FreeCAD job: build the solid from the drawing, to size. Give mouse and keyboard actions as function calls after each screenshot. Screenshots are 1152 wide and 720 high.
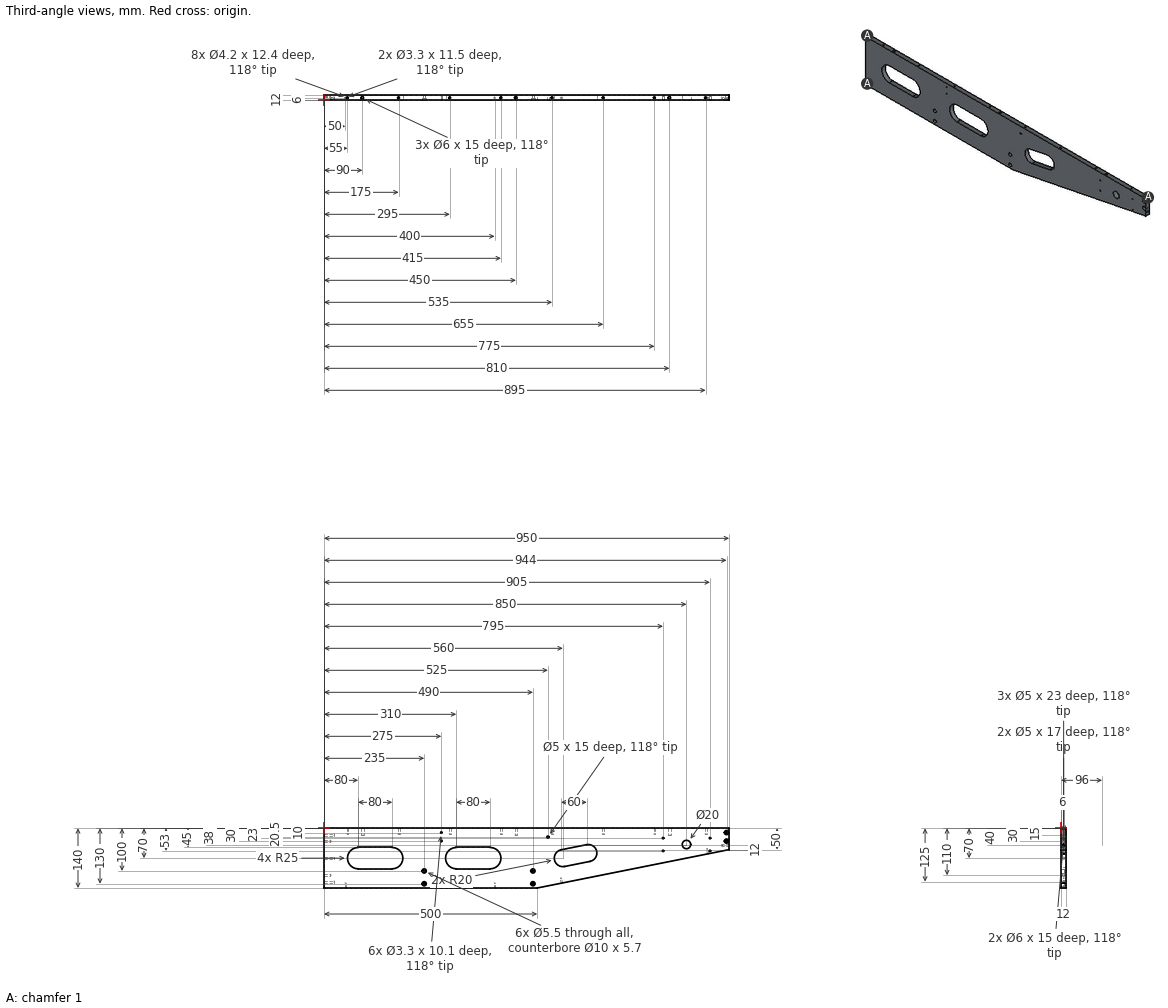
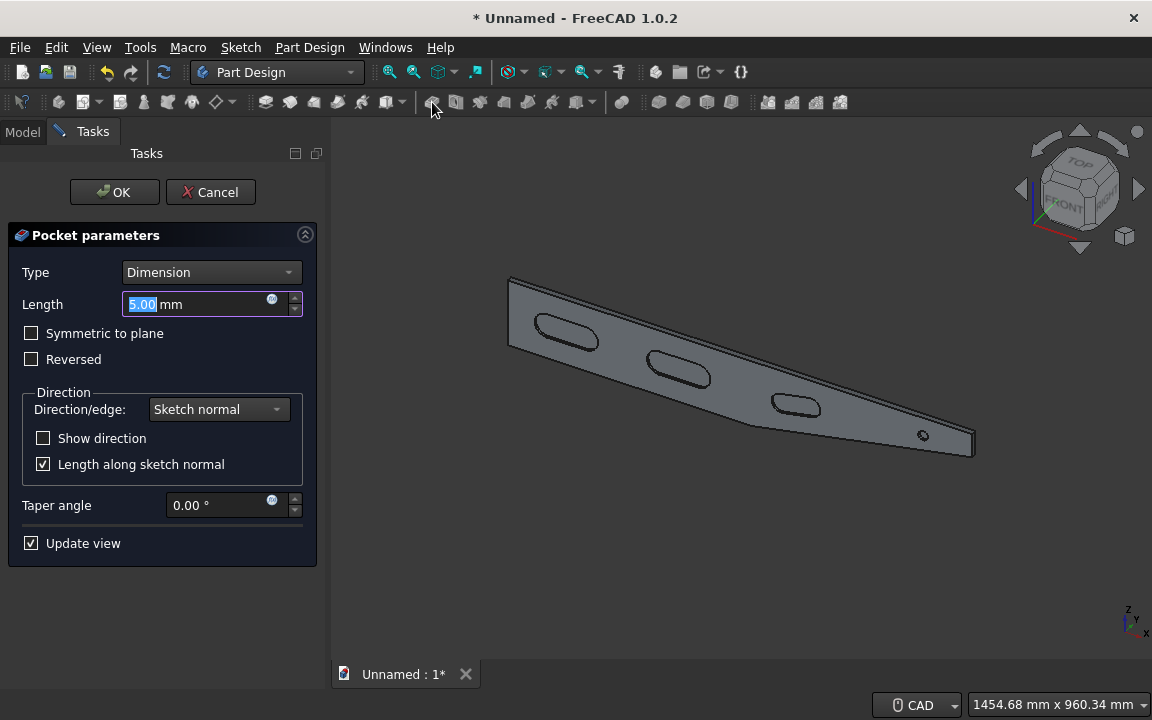
text(12)
key(Tab)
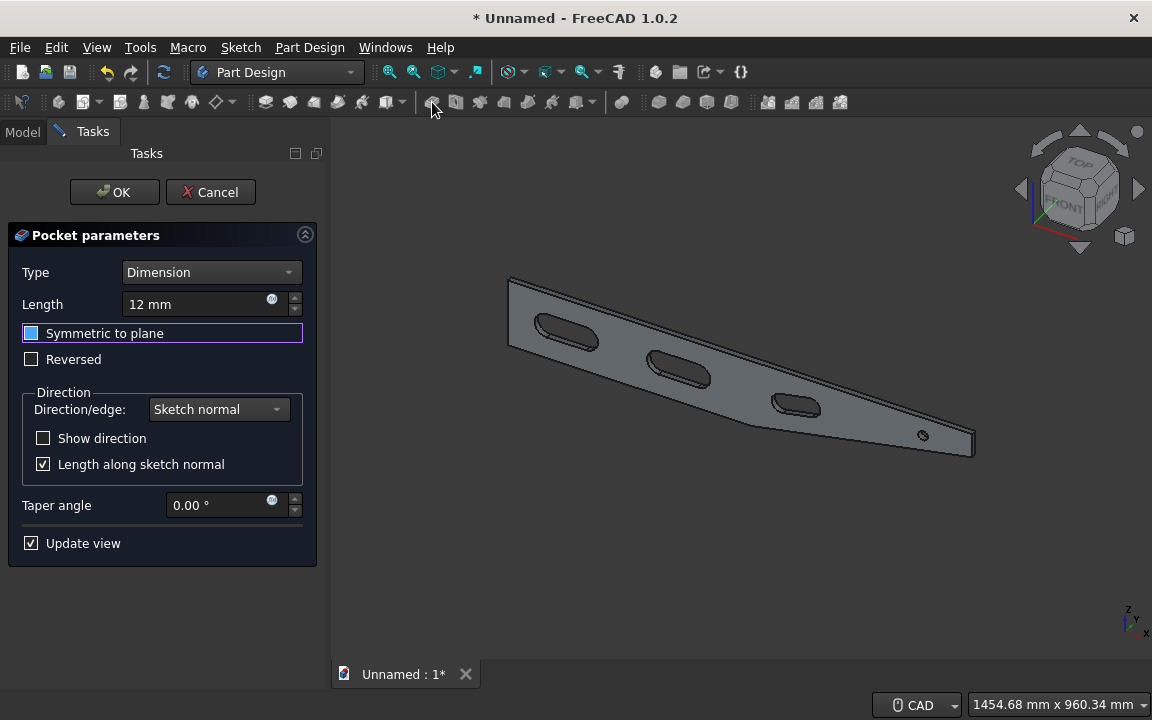
click(115, 192)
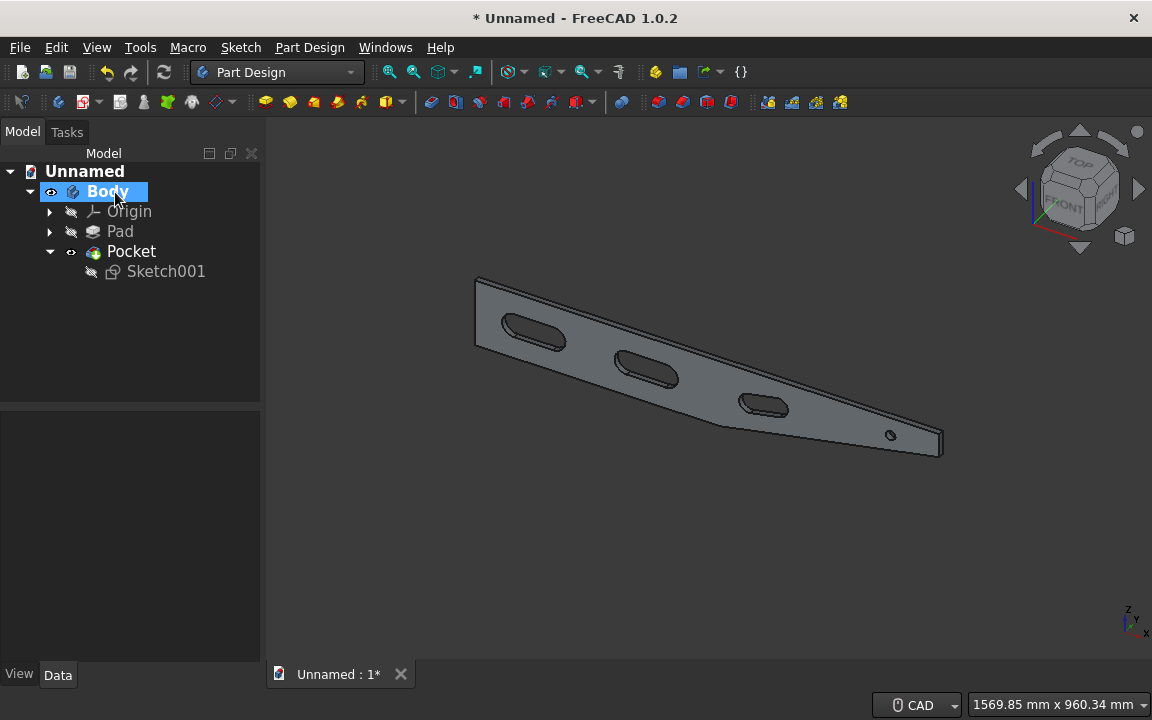
click(84, 102)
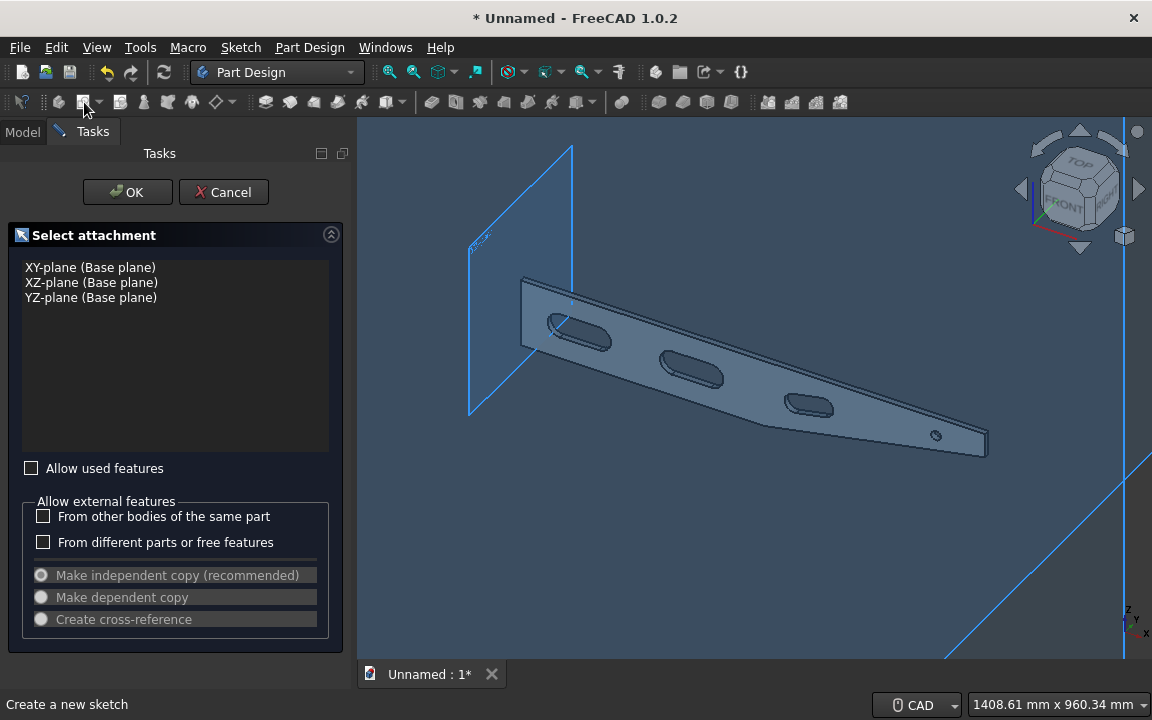
click(82, 282)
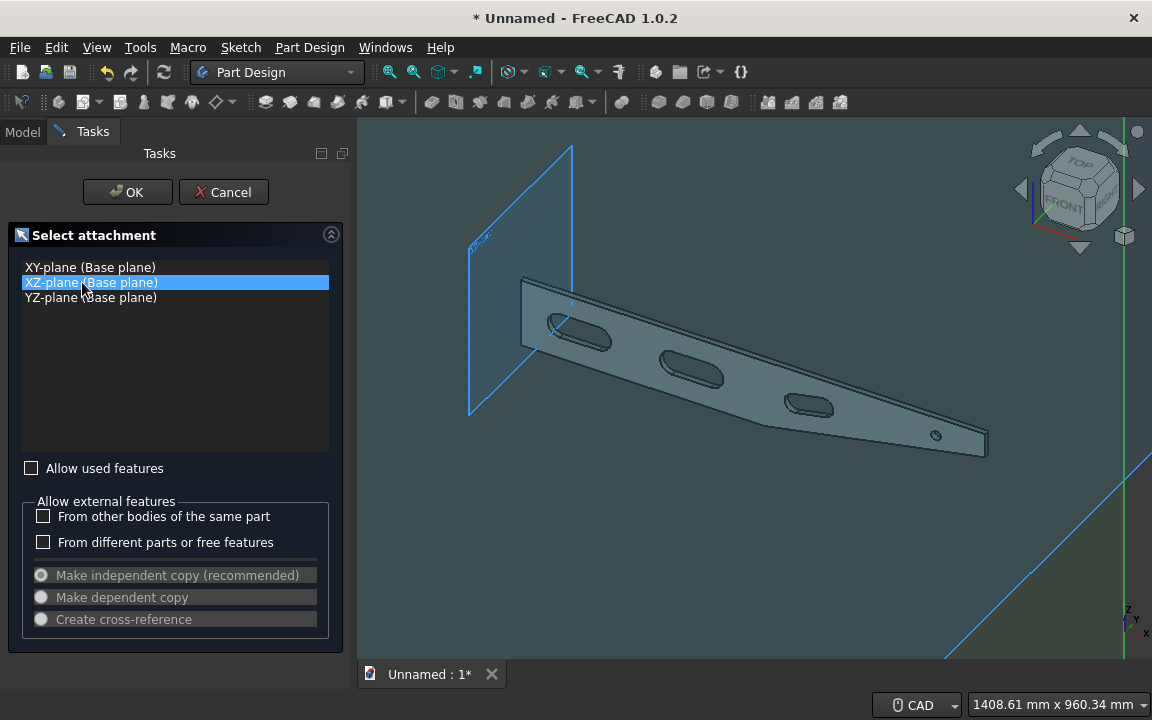
click(128, 192)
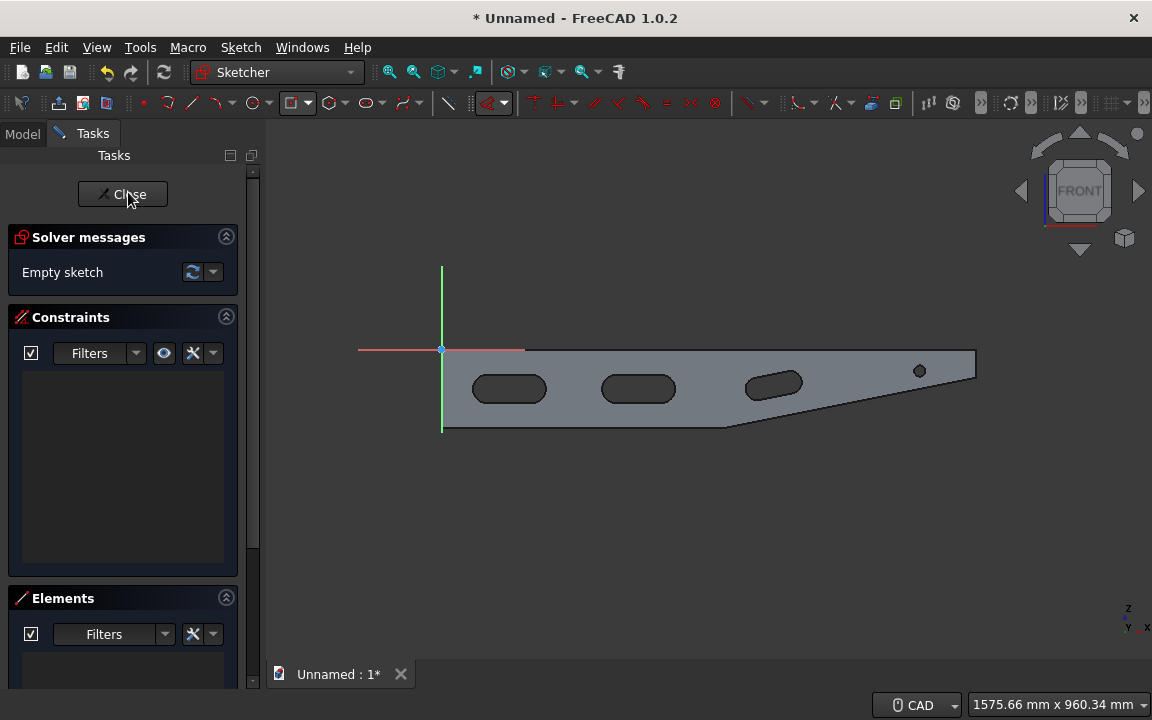
click(254, 104)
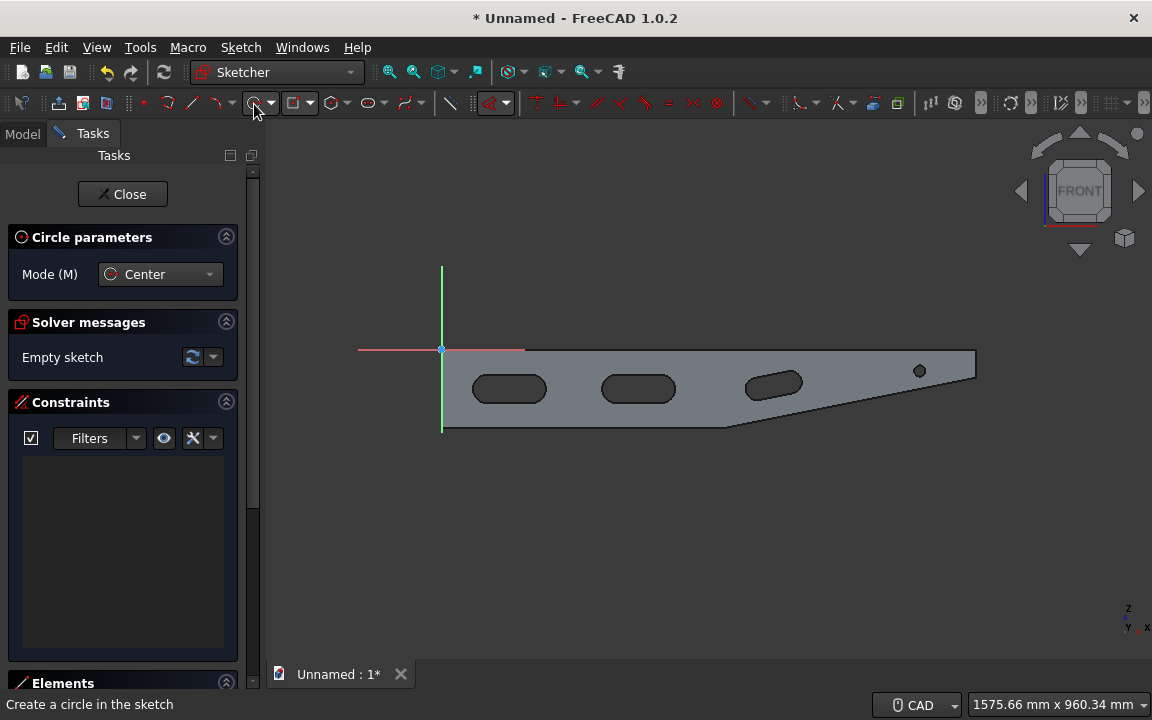
scroll(597, 355, up, 16)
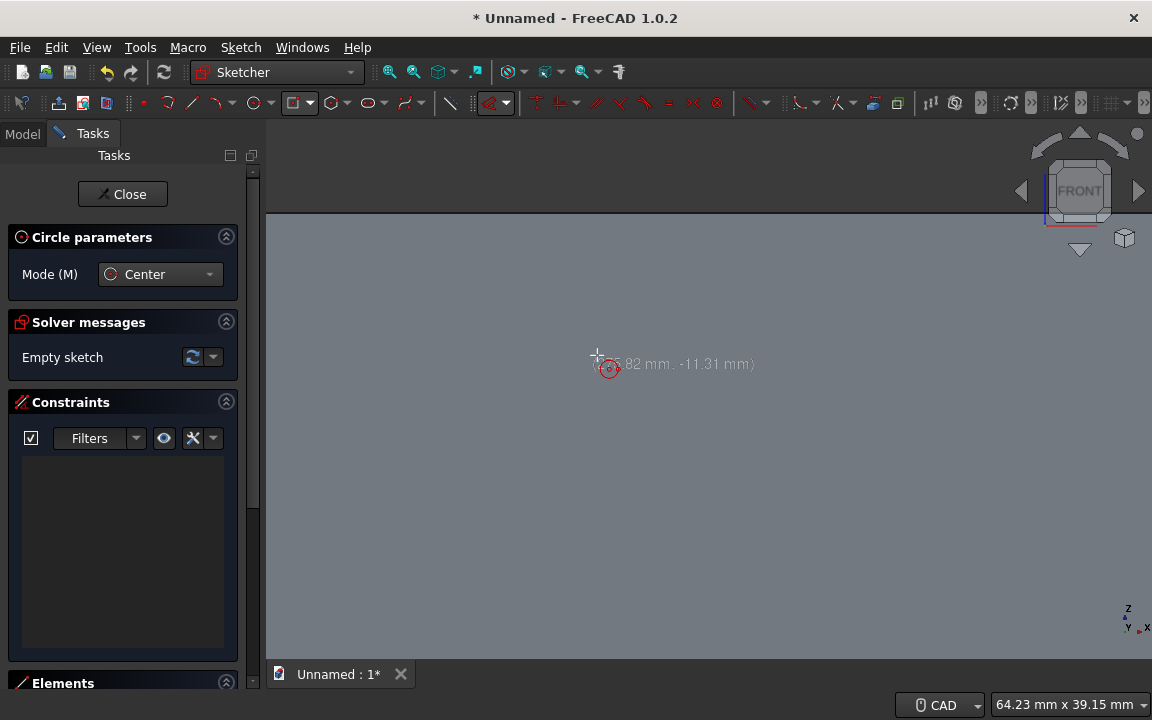
scroll(515, 378, down, 15)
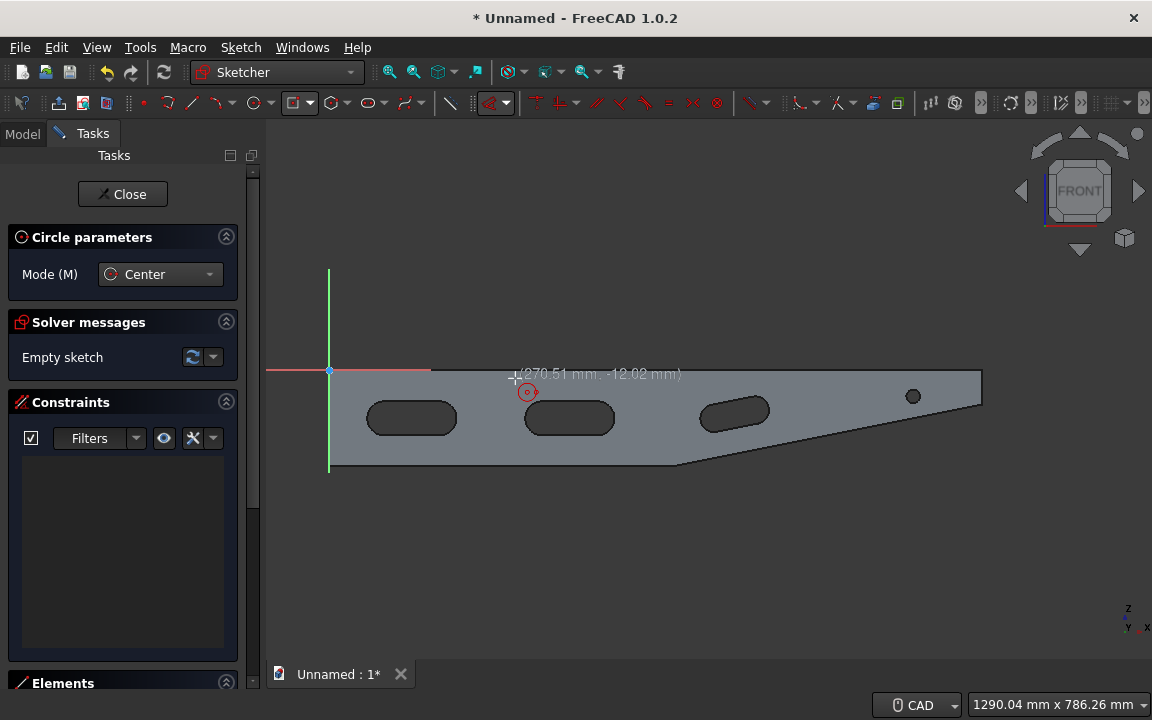
scroll(518, 377, up, 5)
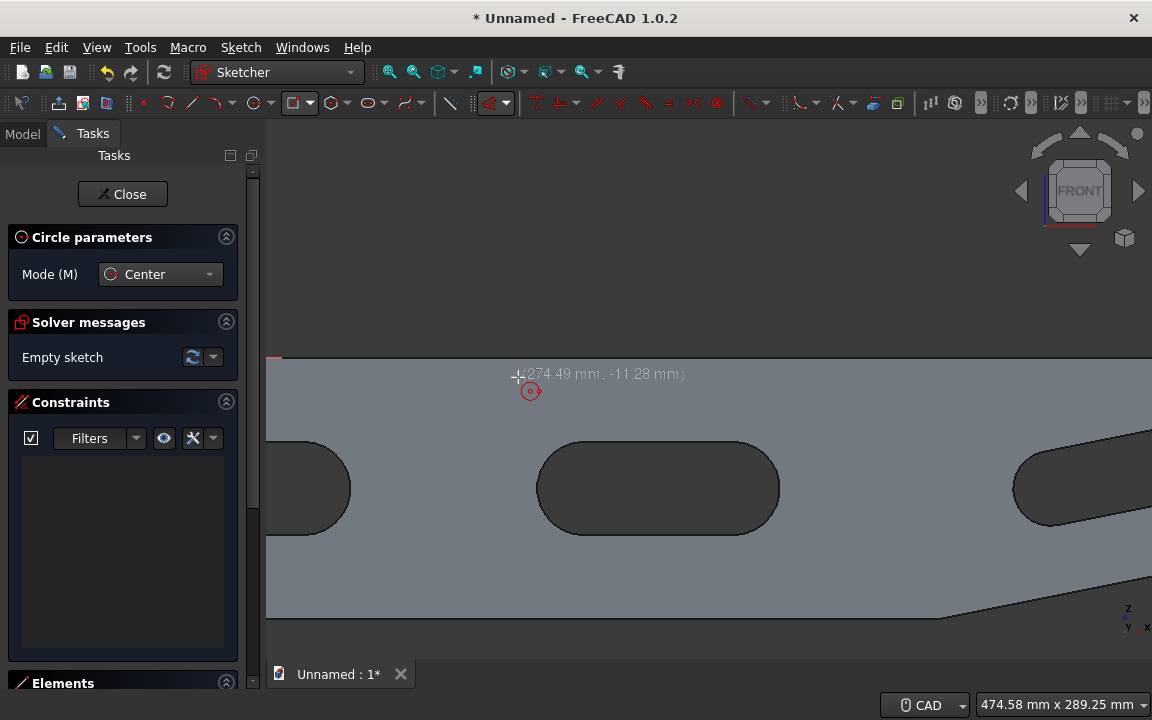
click(518, 376)
move(521, 374)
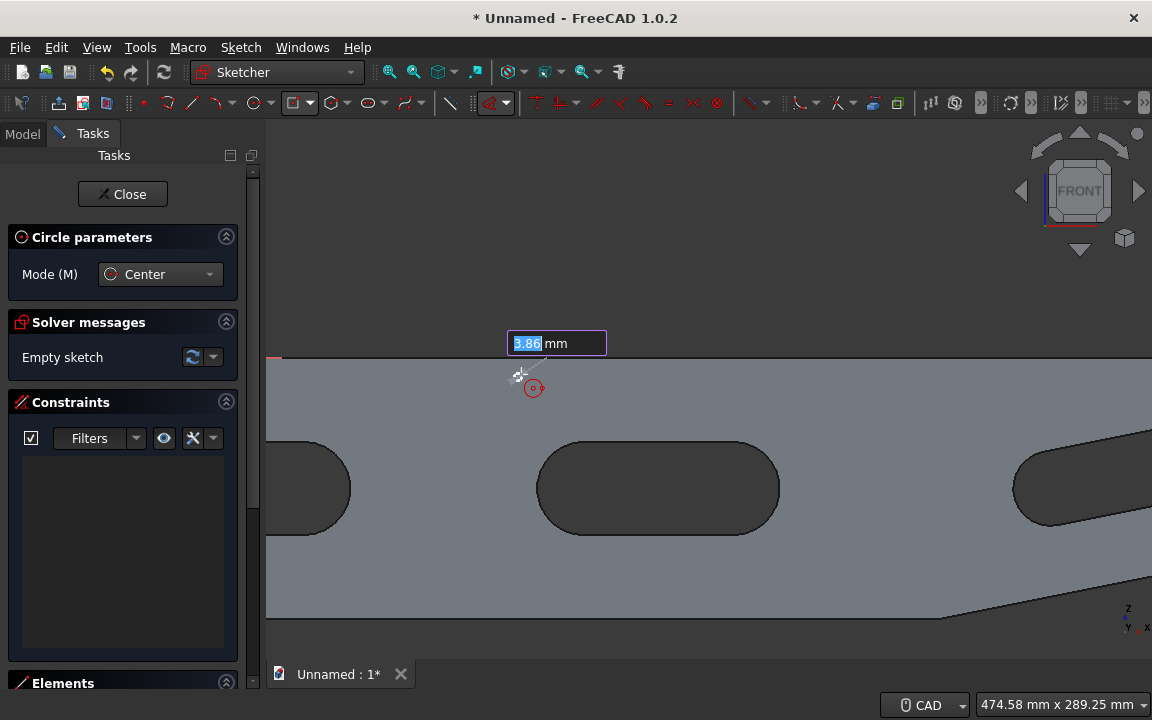
text(3.3)
key(Return)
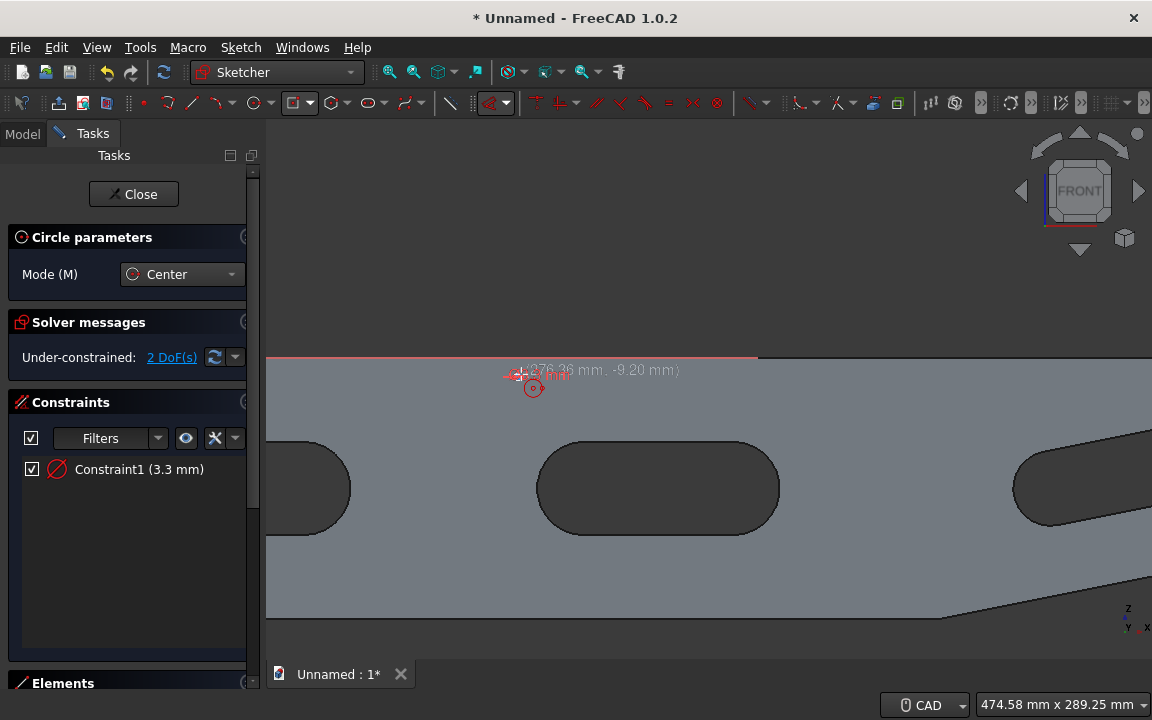
scroll(518, 414, up, 10)